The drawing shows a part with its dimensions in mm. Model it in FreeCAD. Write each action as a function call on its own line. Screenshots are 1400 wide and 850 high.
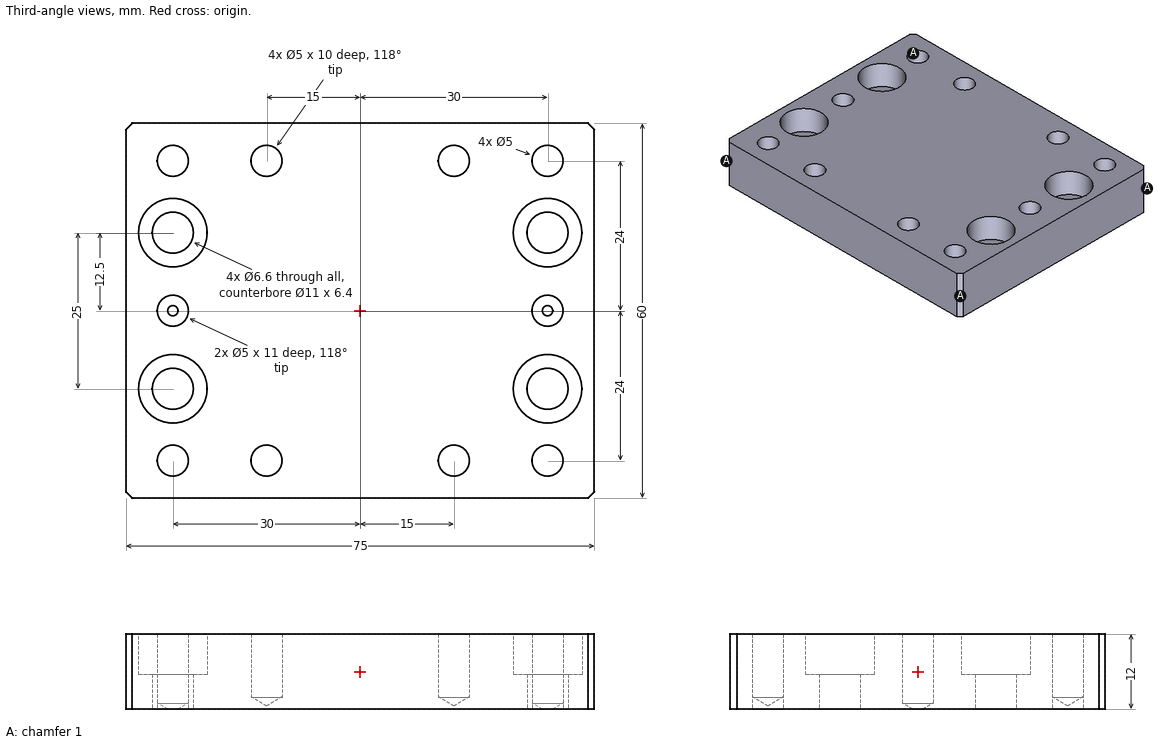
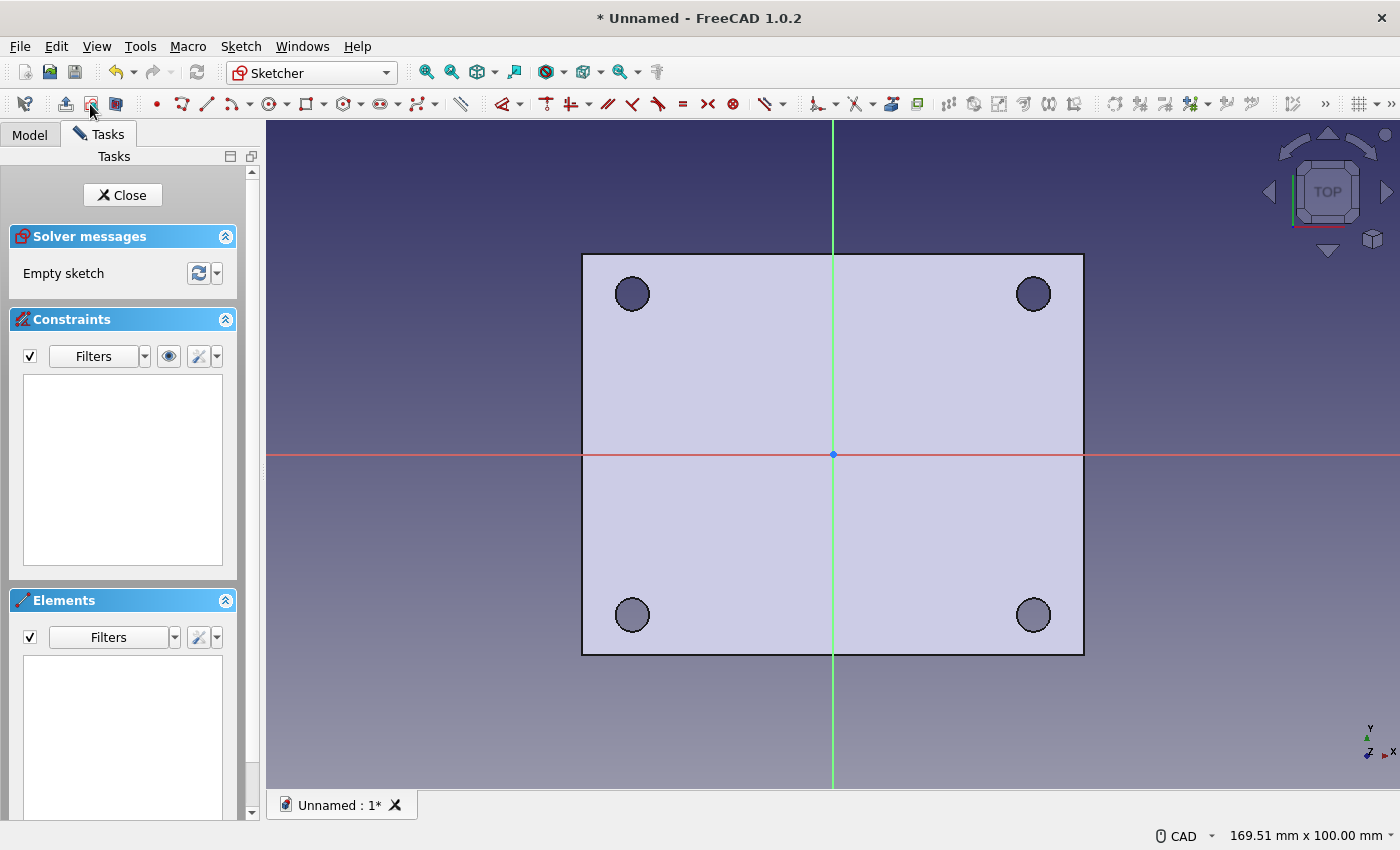
scroll(972, 455, up, 2)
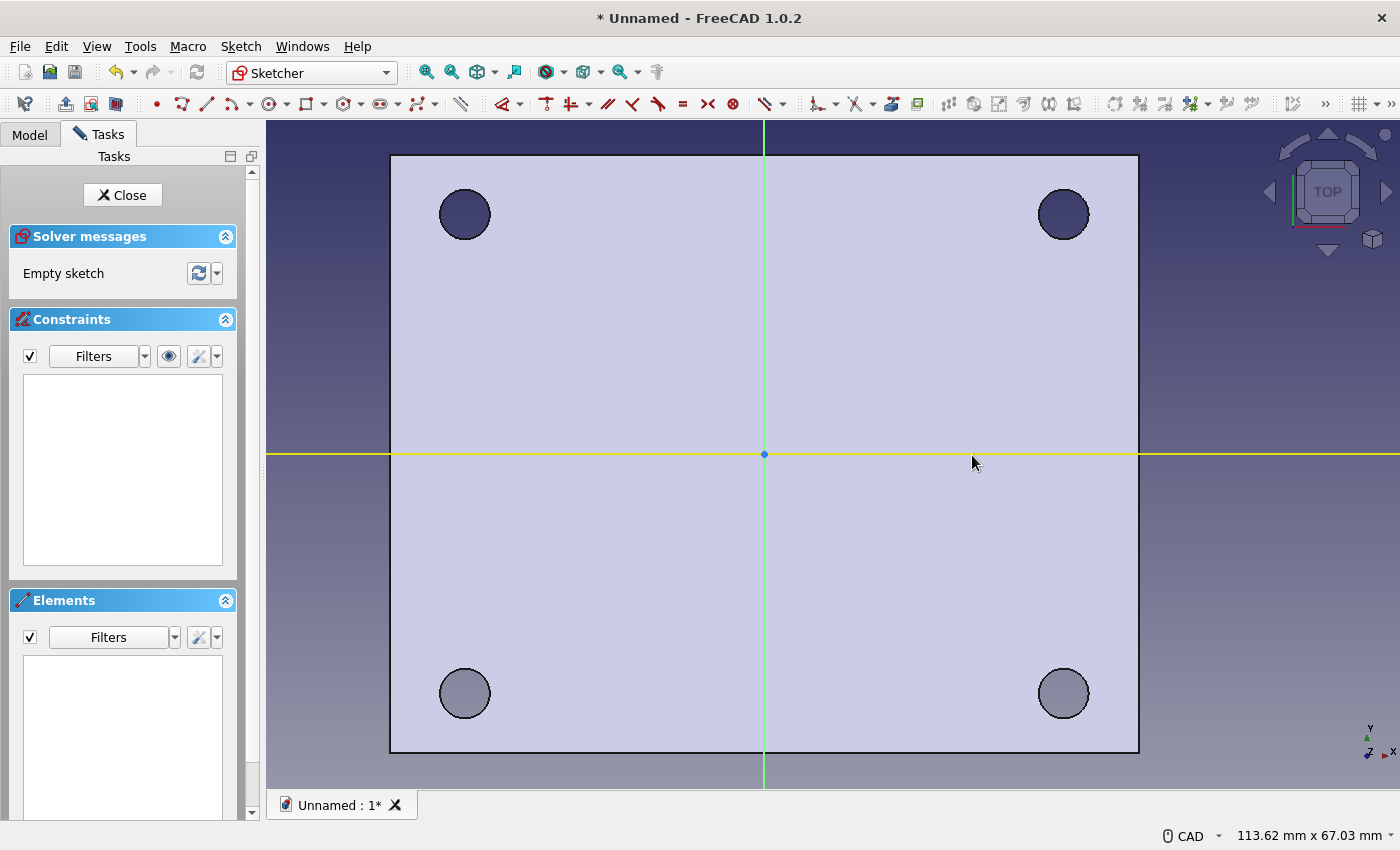
key(g)
key(c)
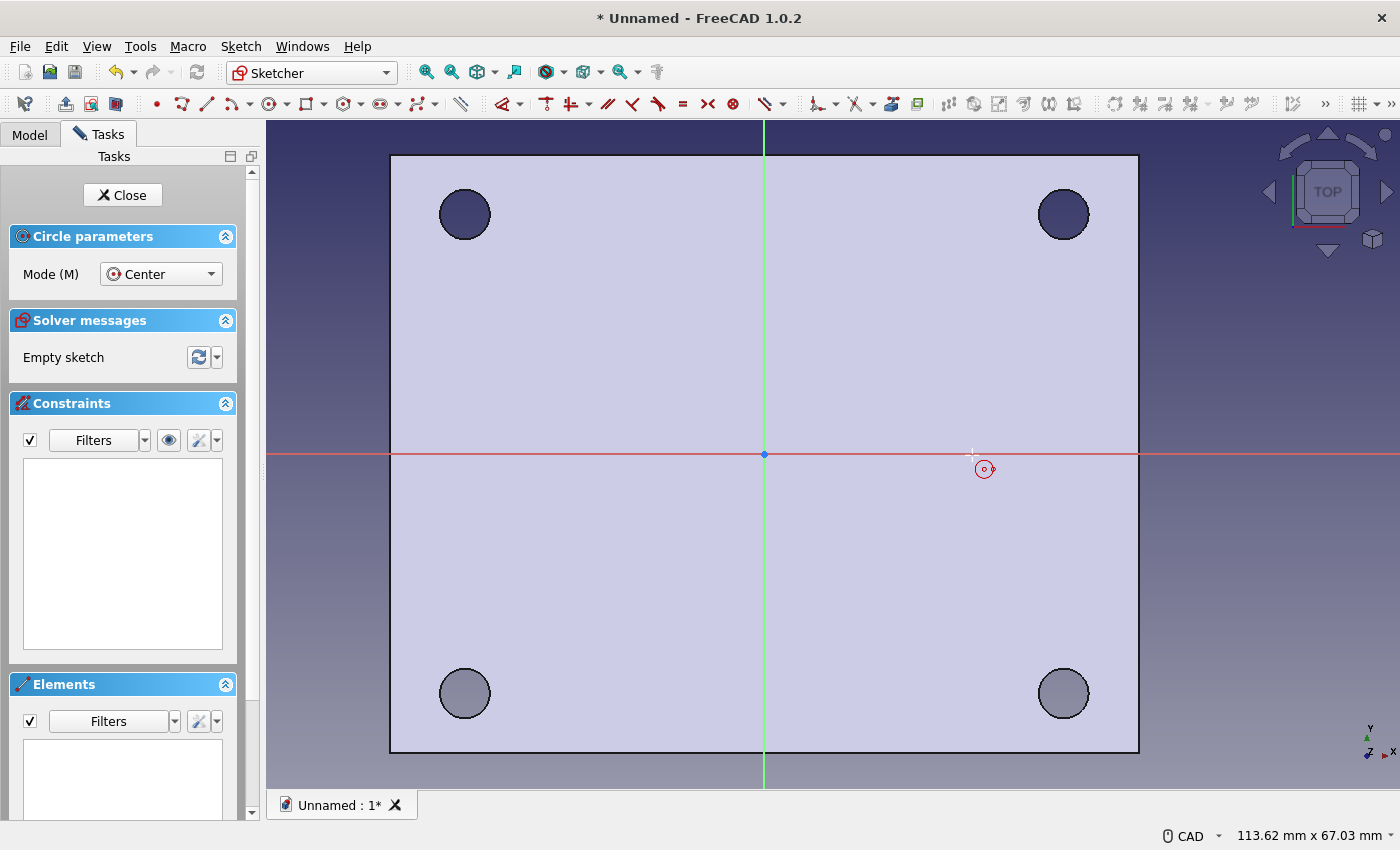
click(465, 329)
click(488, 306)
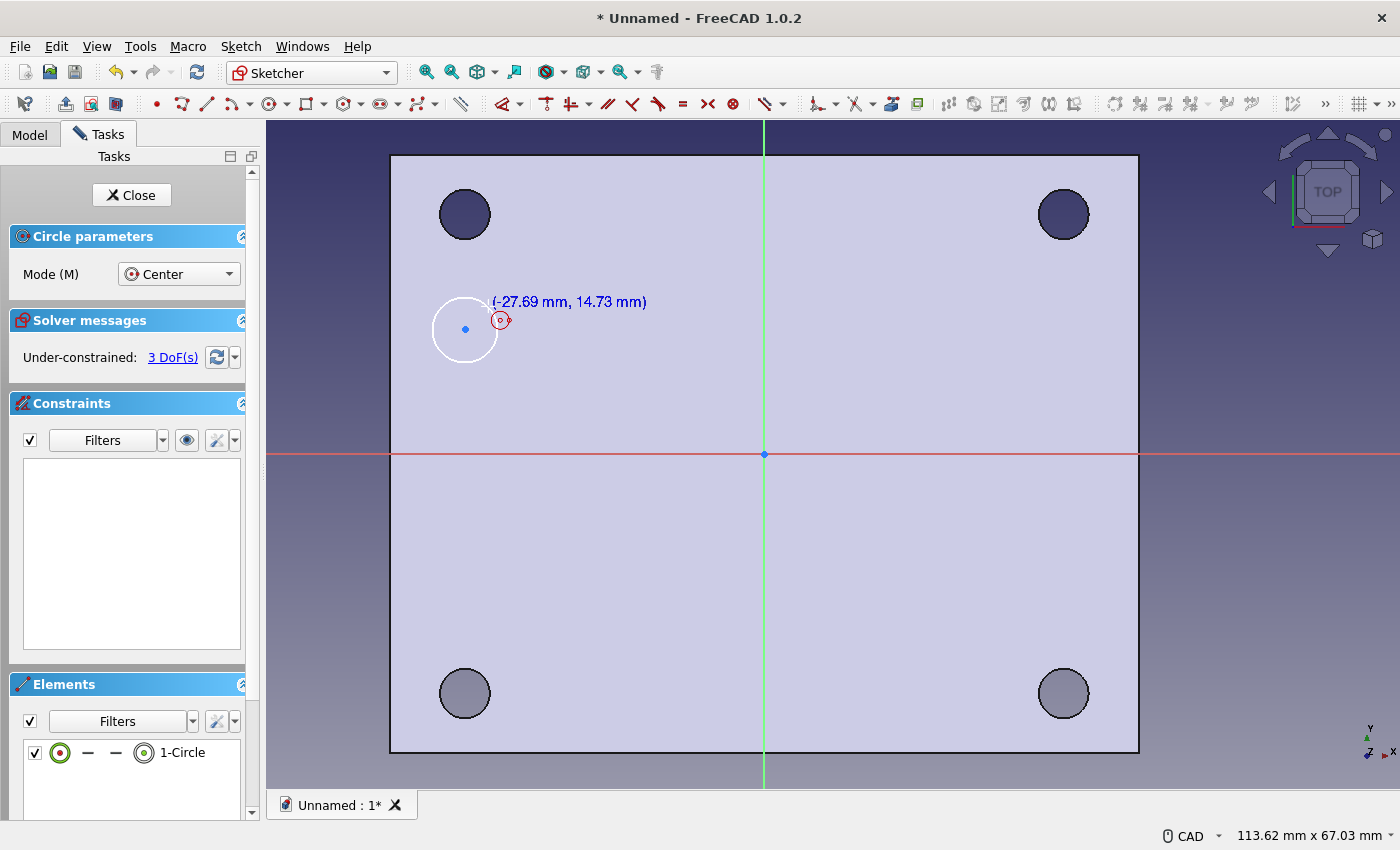
click(1064, 329)
click(1087, 306)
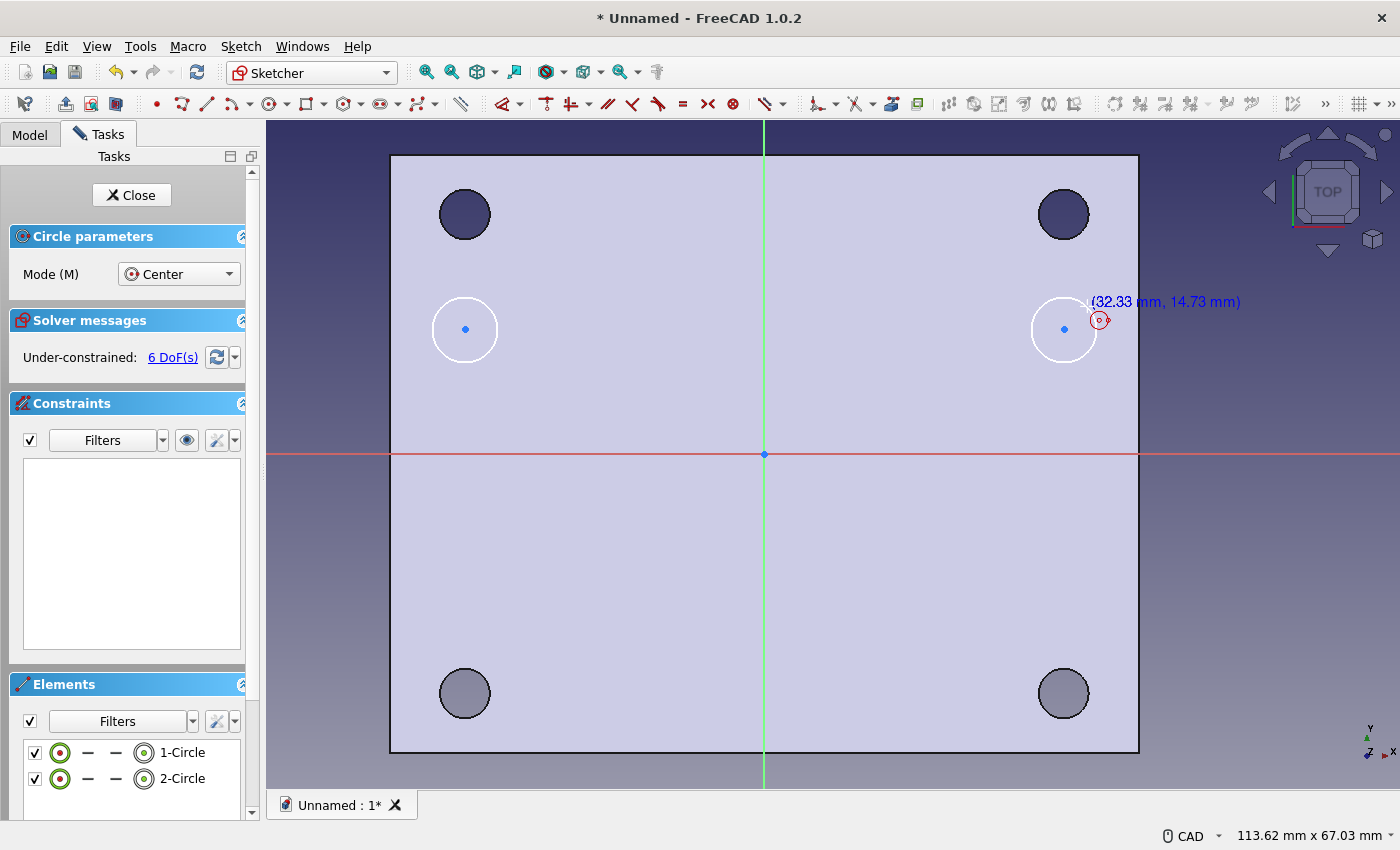
click(465, 579)
click(488, 555)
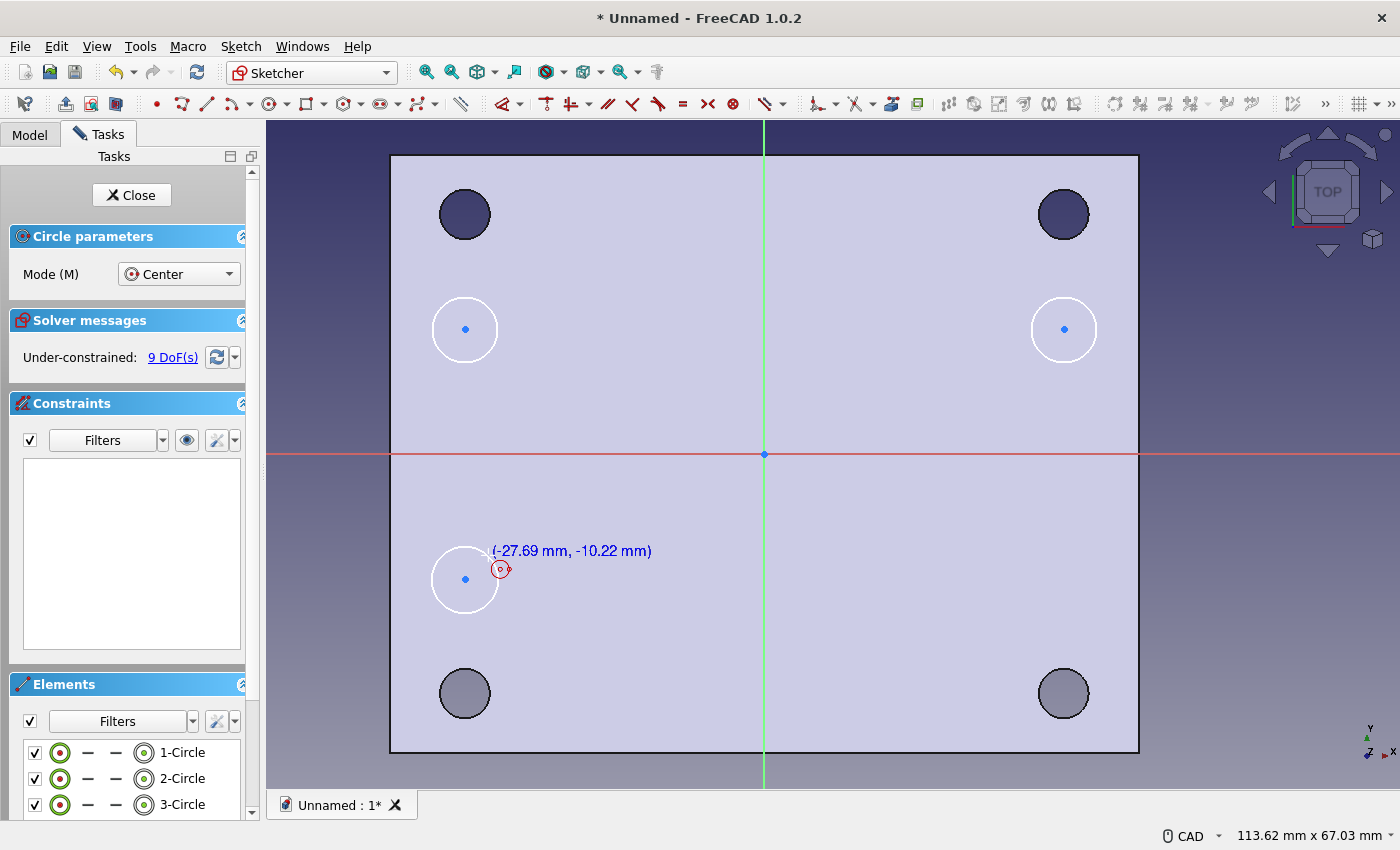
click(1064, 579)
click(1087, 555)
key(Escape)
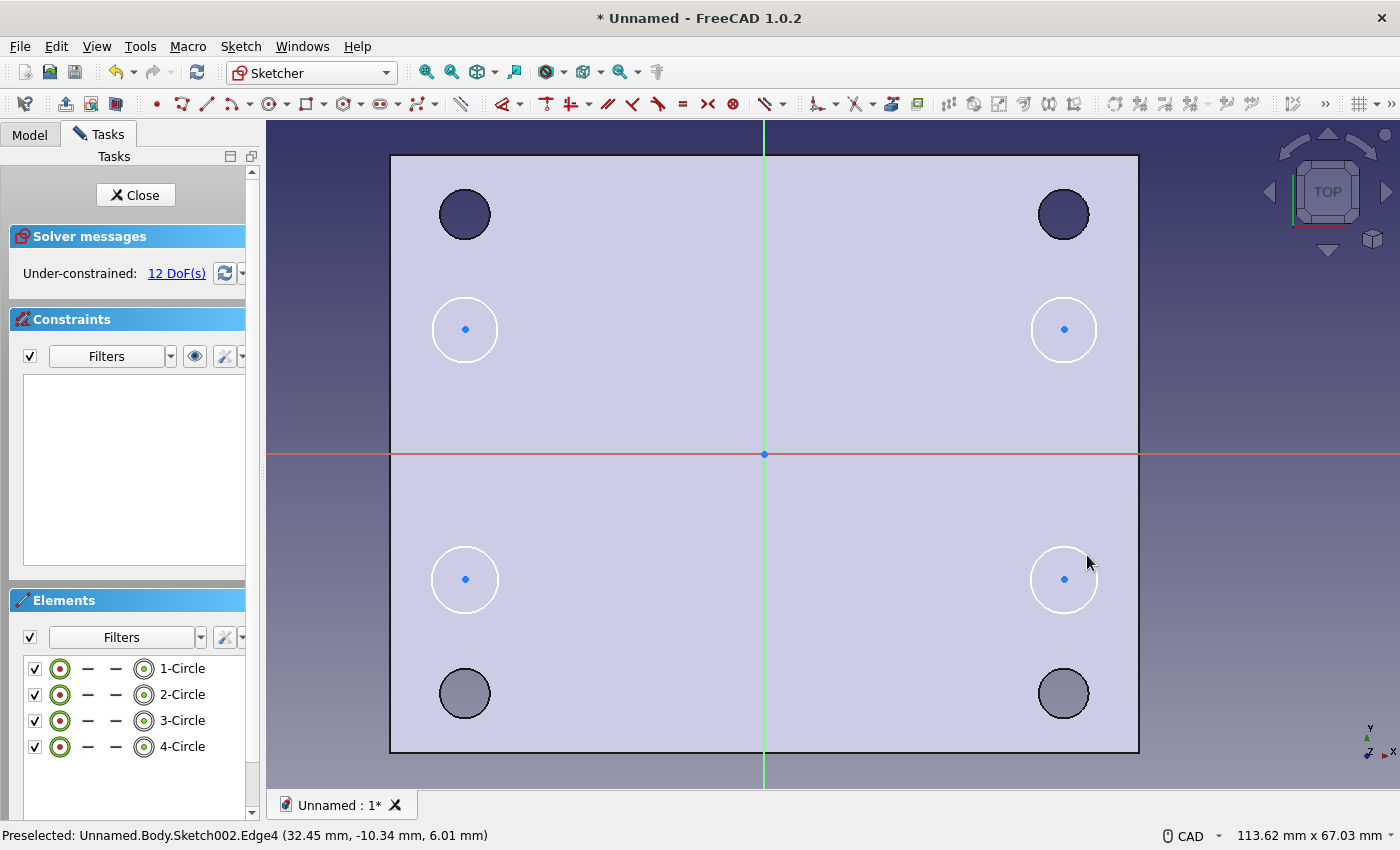
click(488, 307)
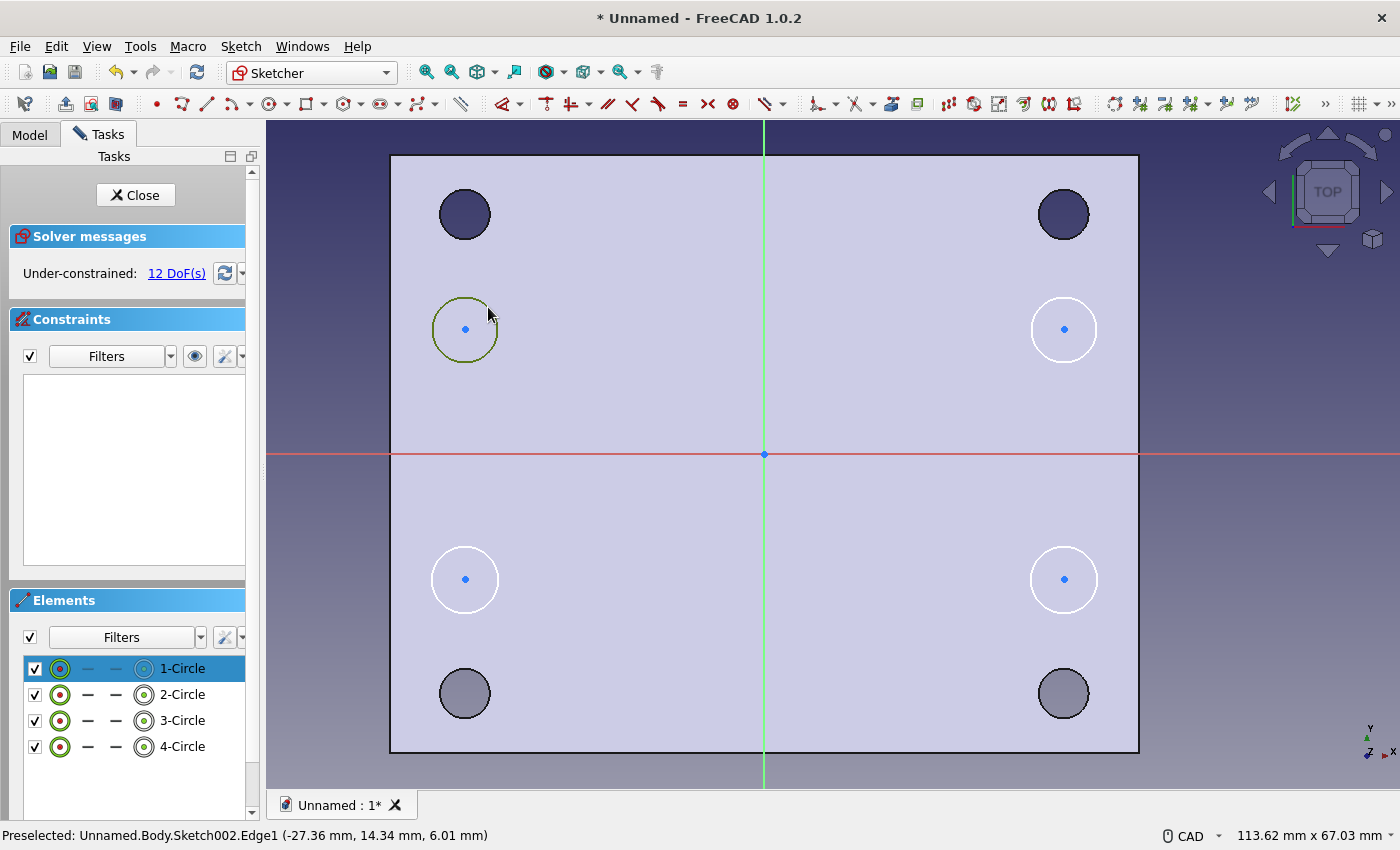
click(1087, 307)